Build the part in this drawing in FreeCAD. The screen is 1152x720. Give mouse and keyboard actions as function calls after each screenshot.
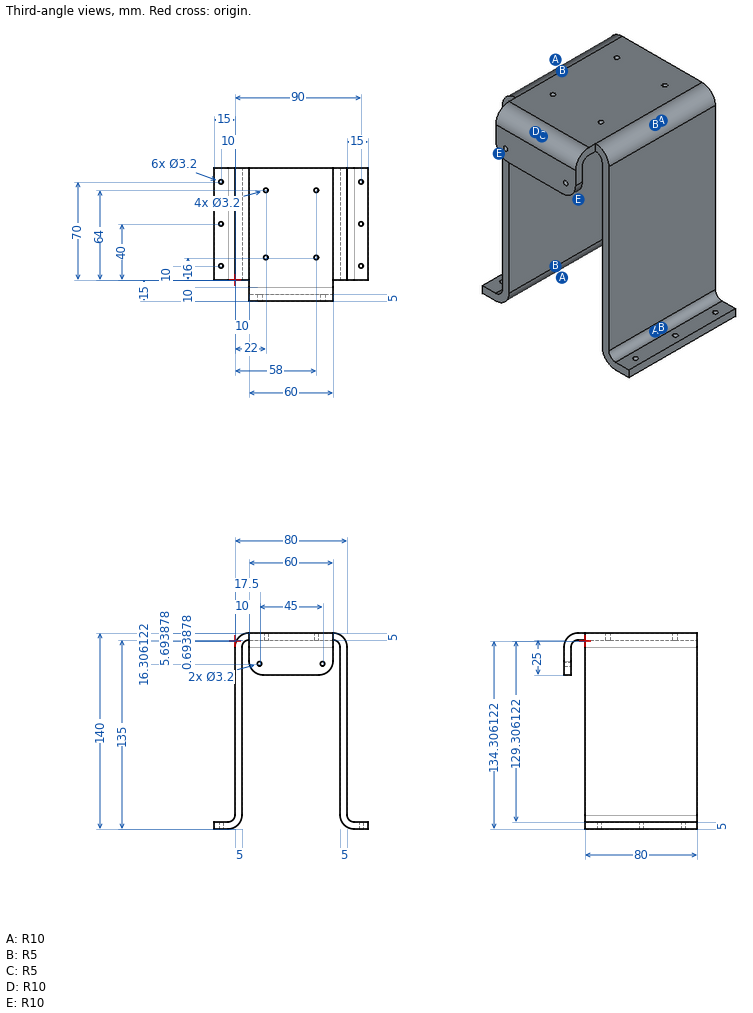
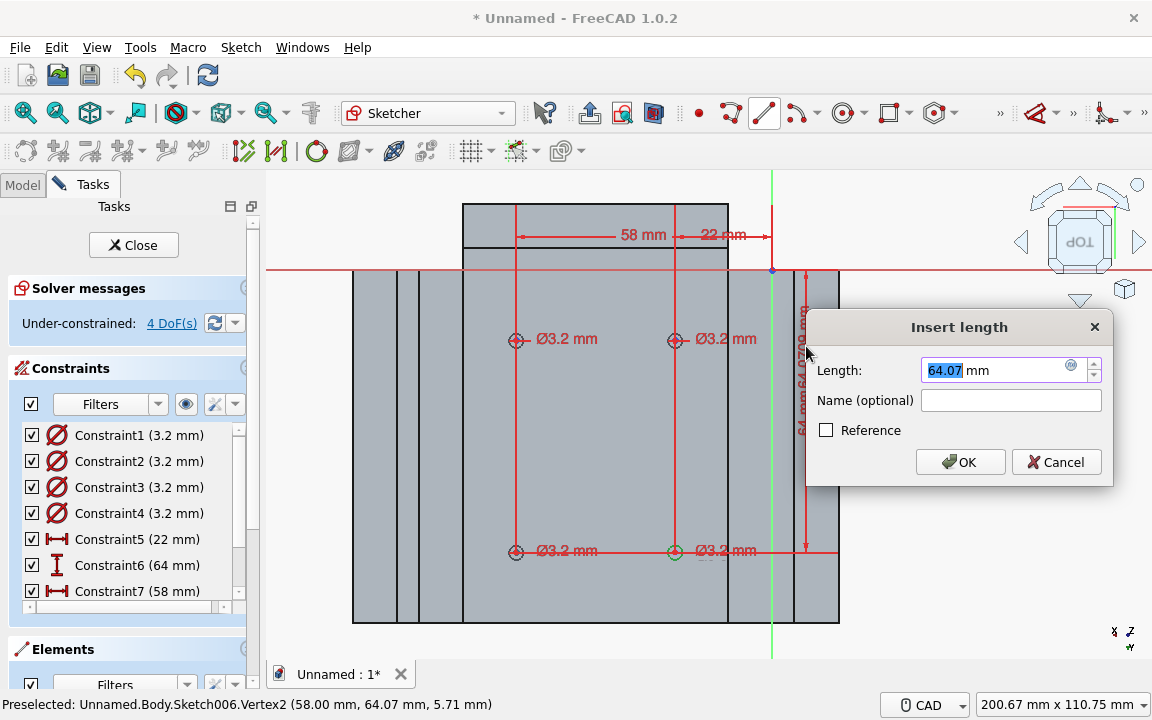
text(64)
key(Return)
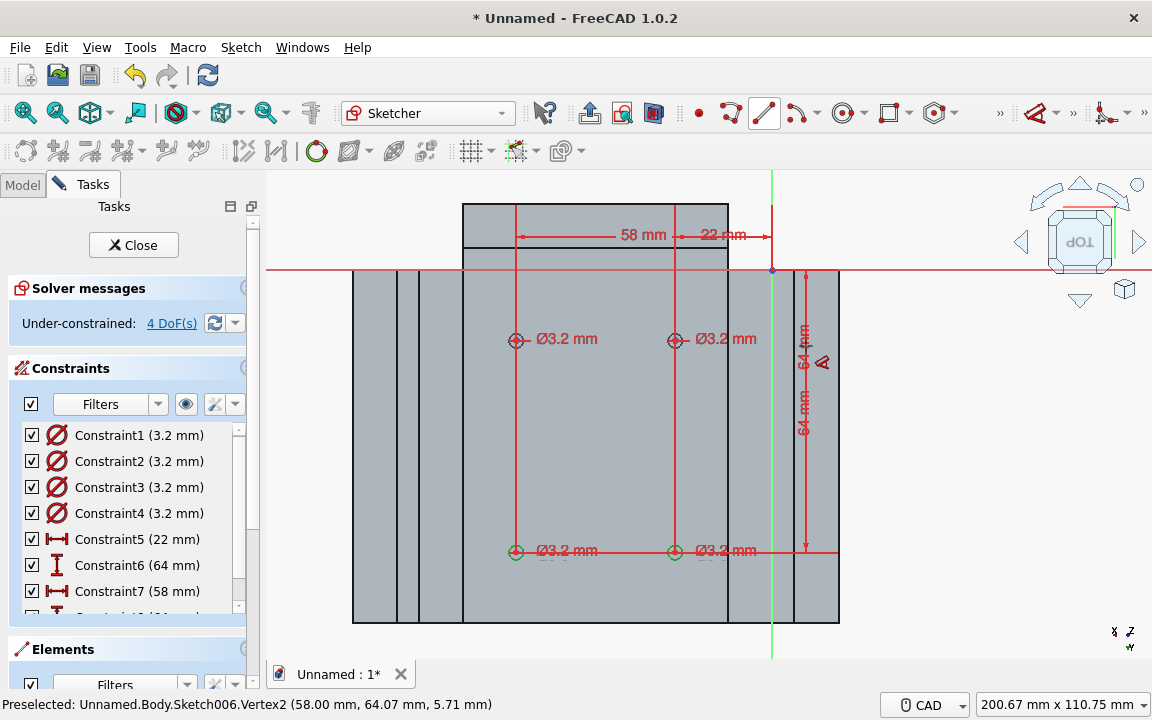
click(516, 341)
click(555, 236)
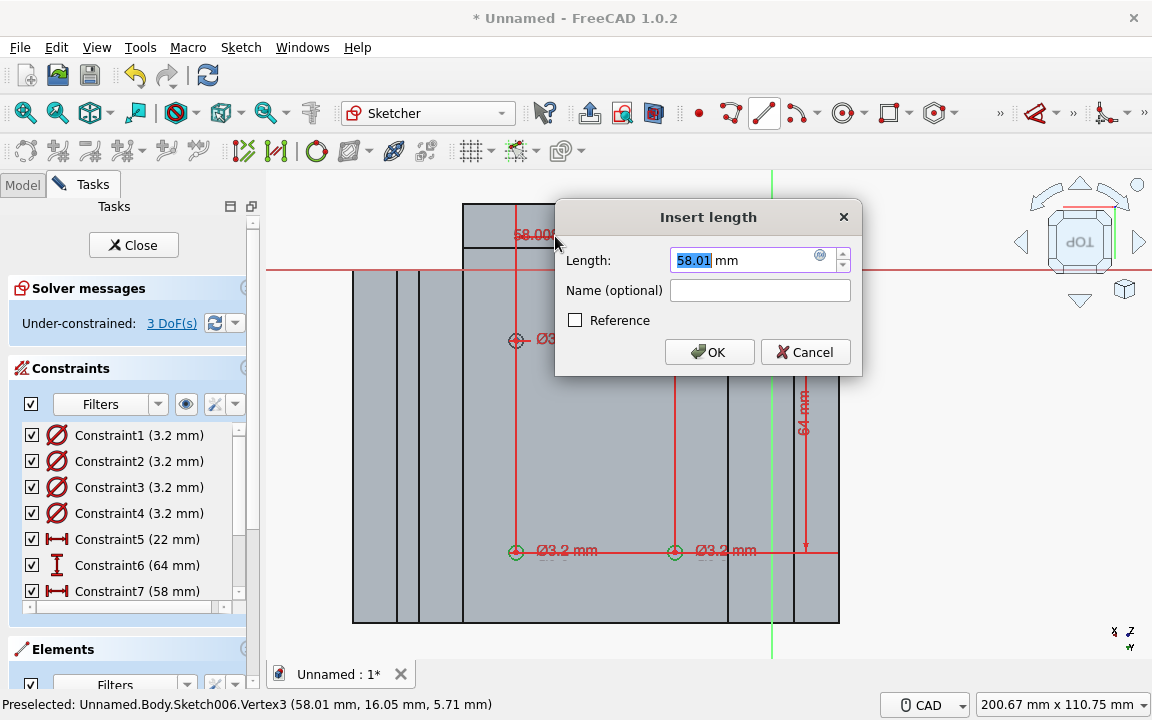
text(58)
key(Return)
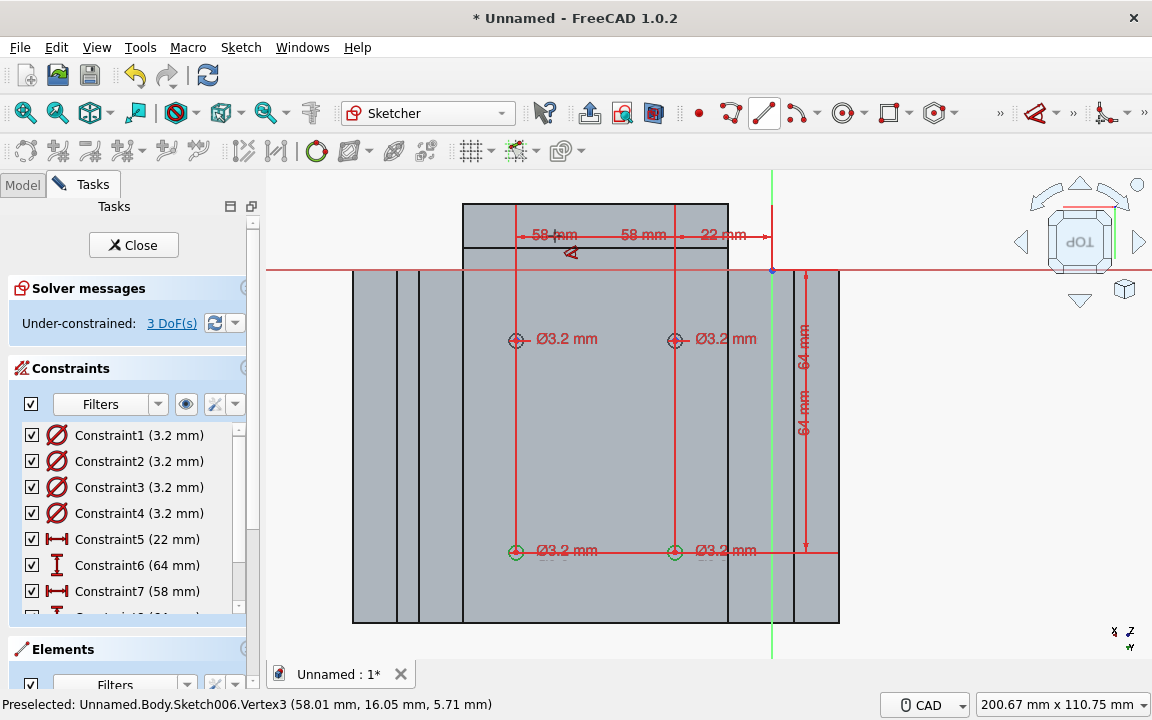
click(516, 341)
click(806, 306)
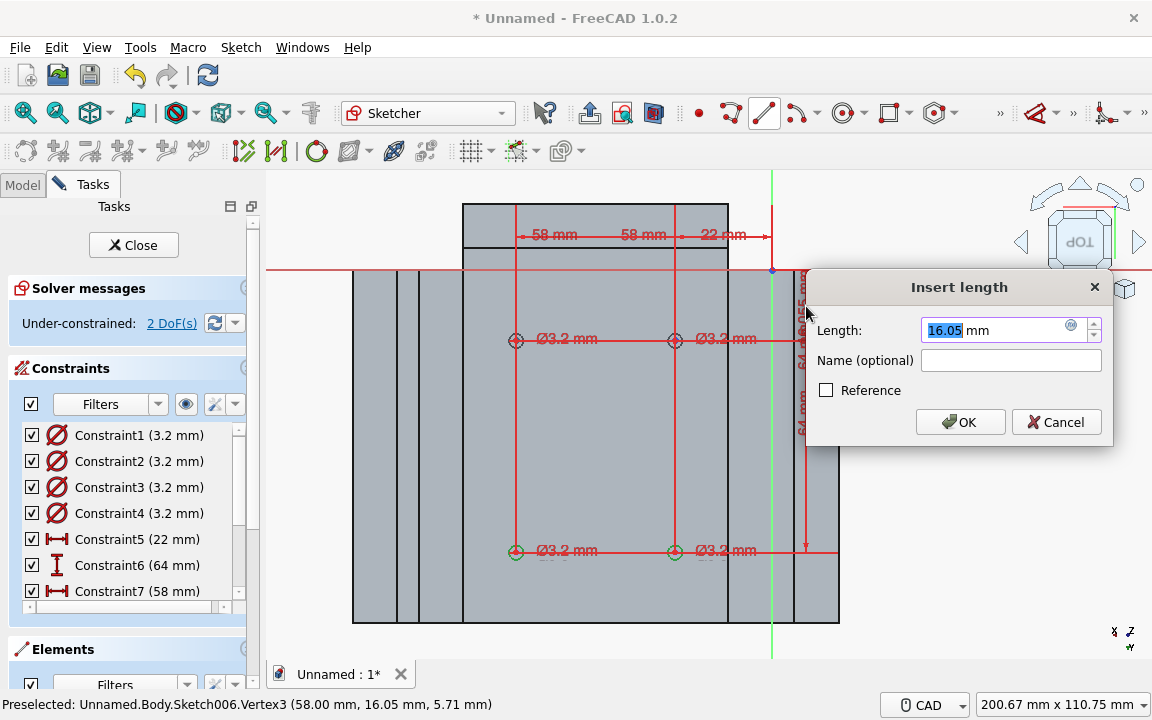
text(16)
key(Return)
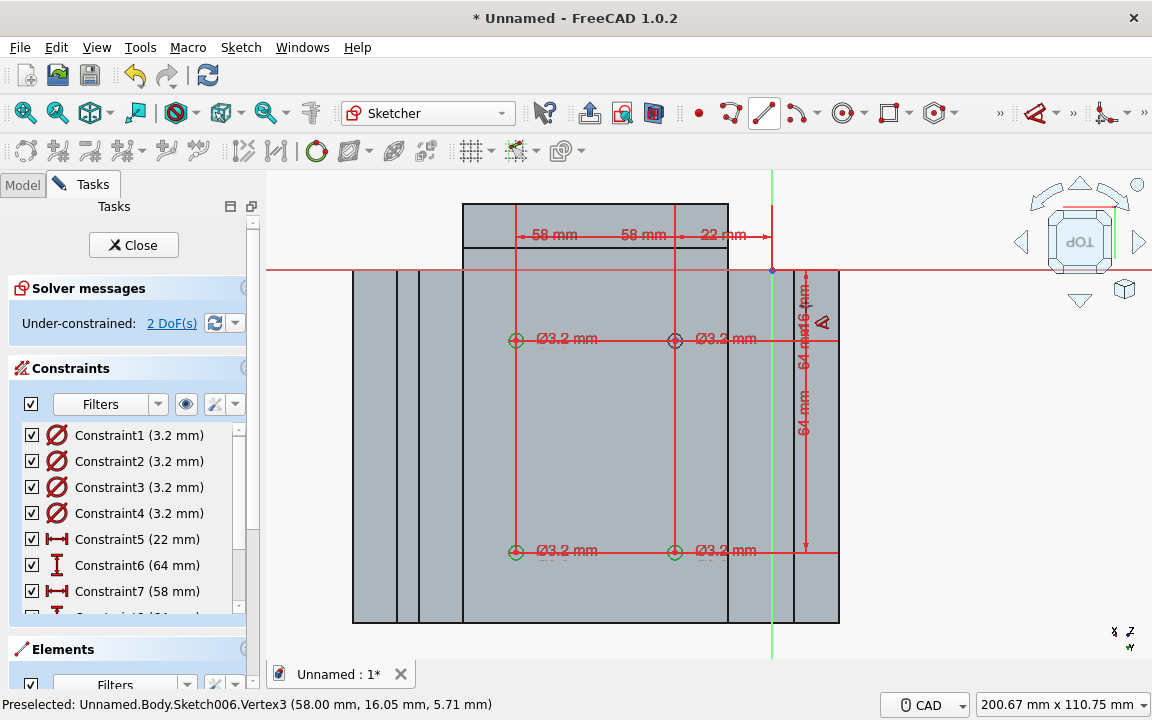
click(675, 341)
click(724, 375)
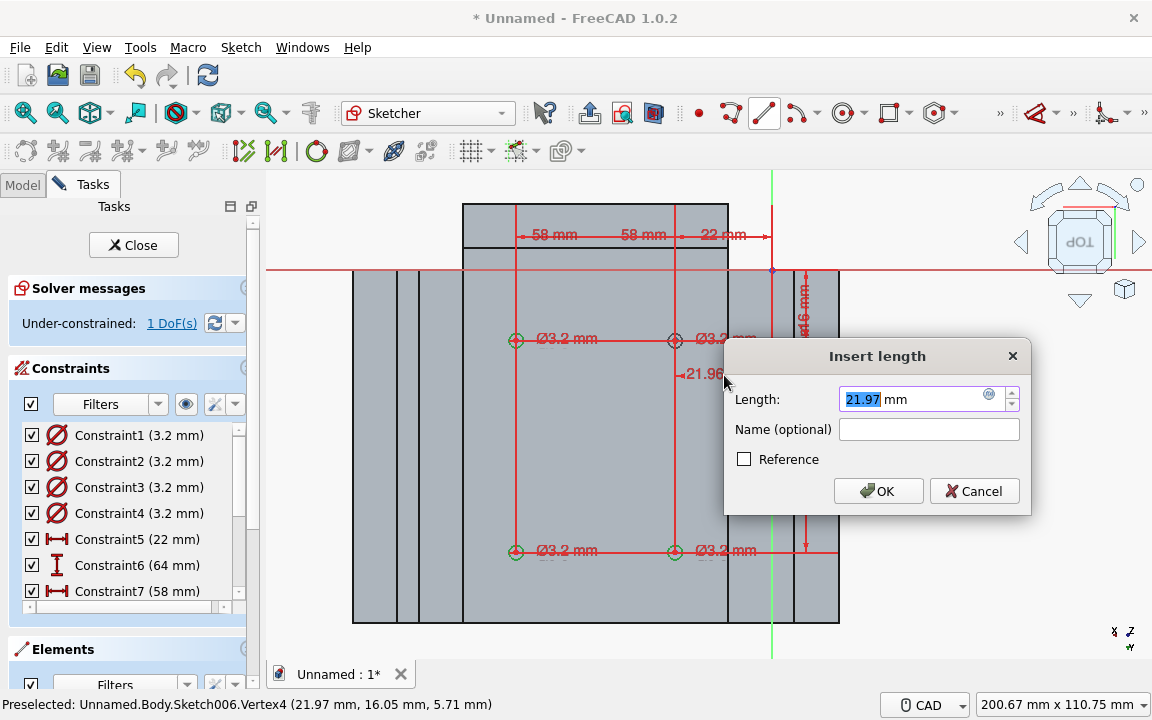
text(22)
key(Return)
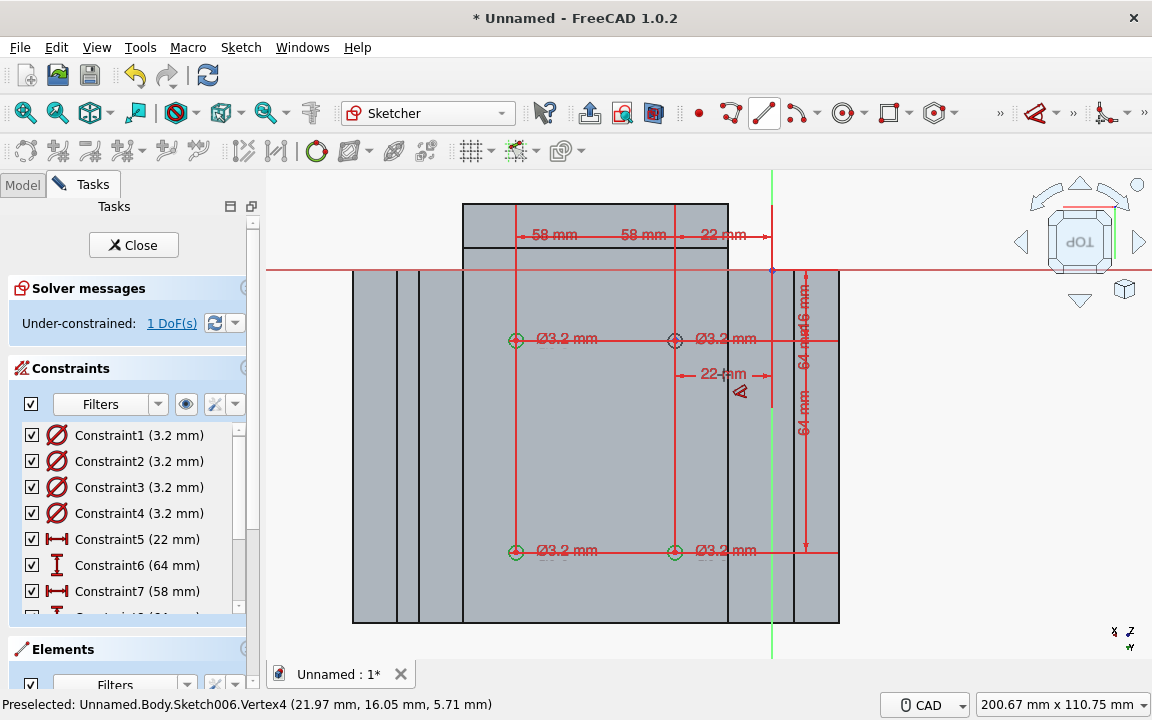
click(675, 341)
click(641, 306)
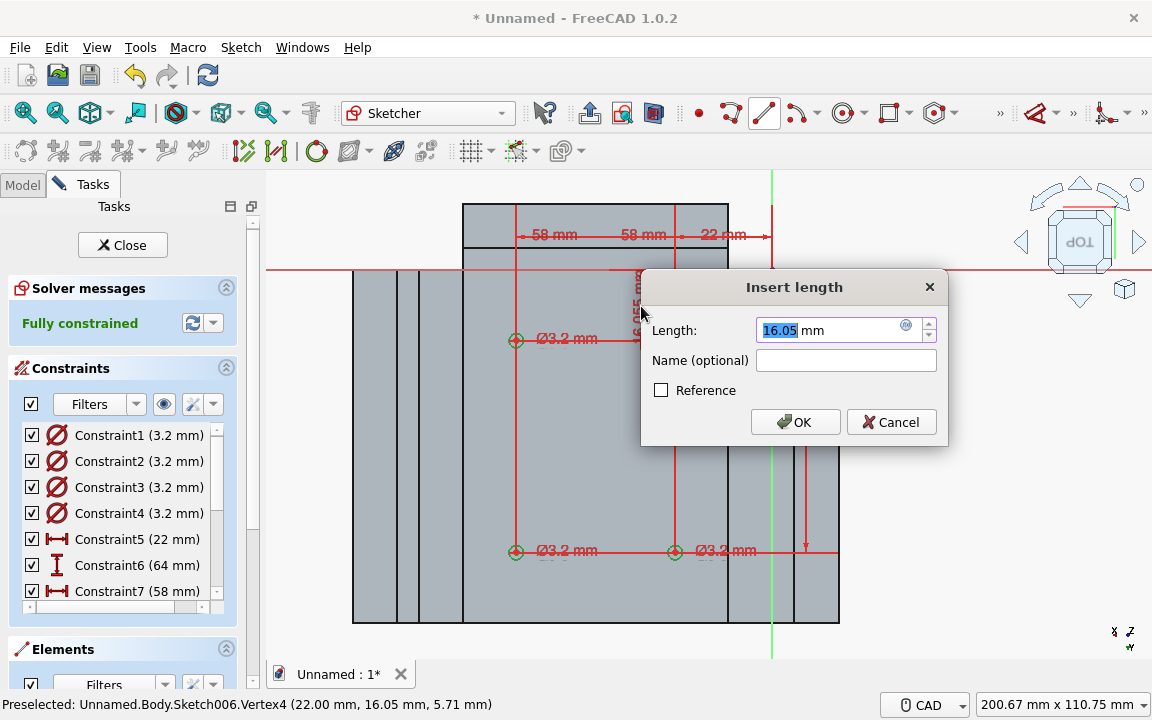
text(16)
key(Return)
key(Escape)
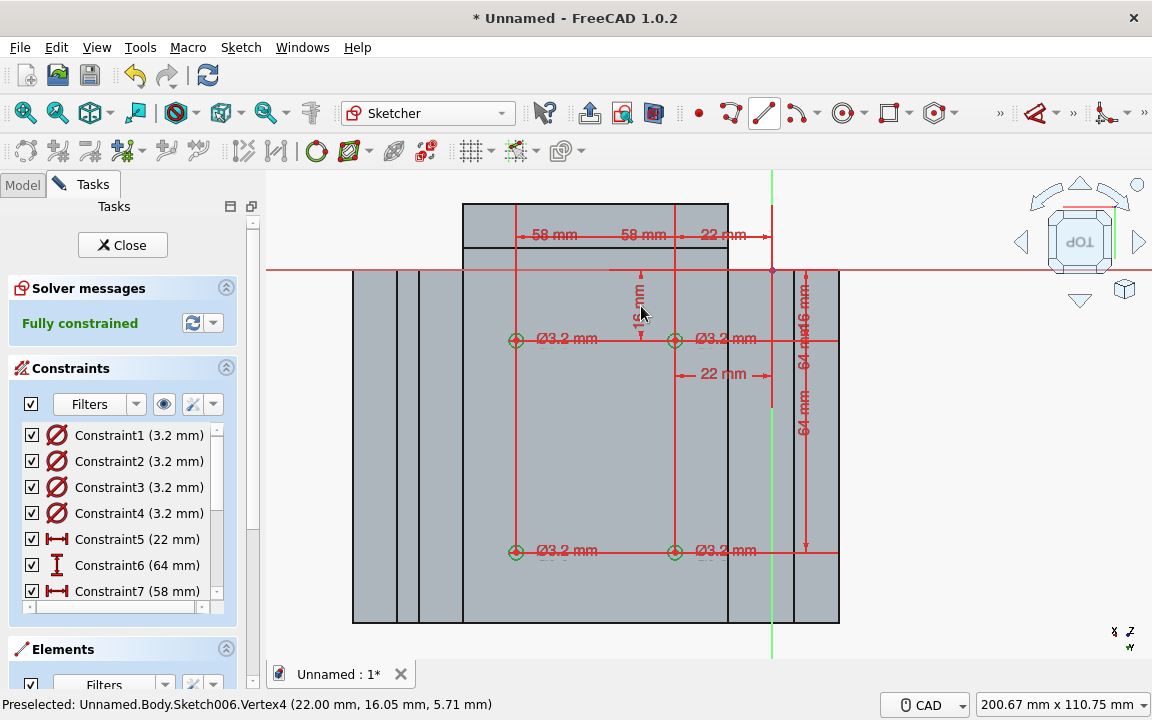
click(123, 245)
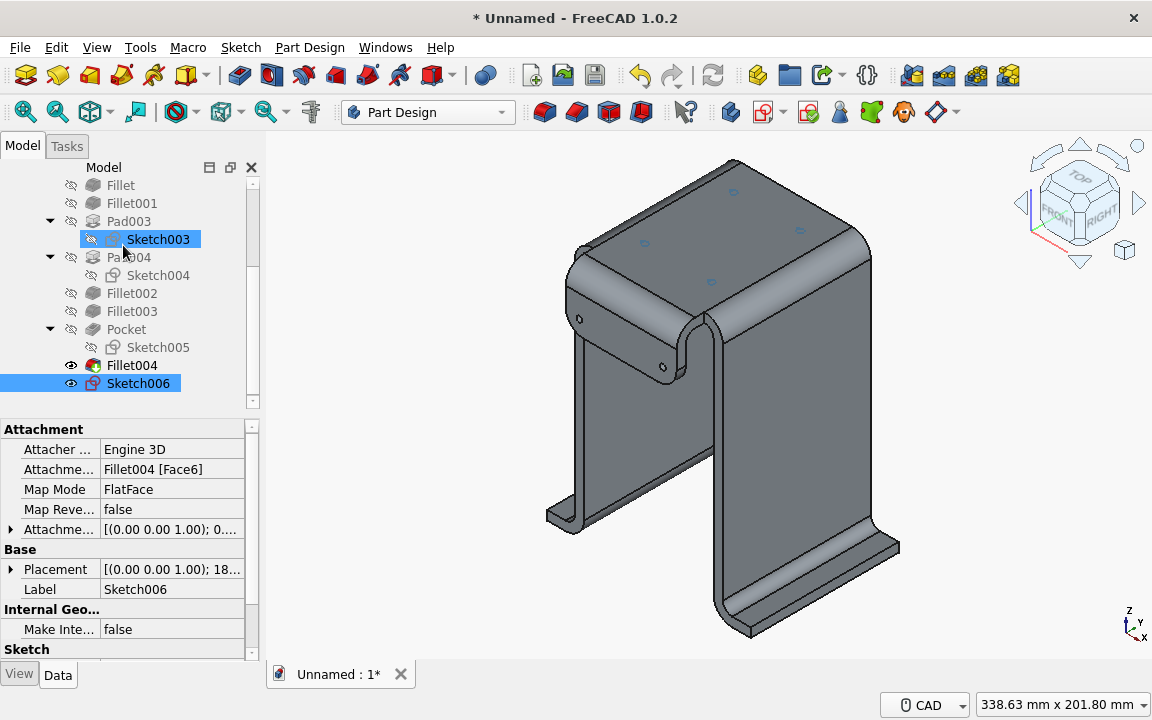
click(240, 76)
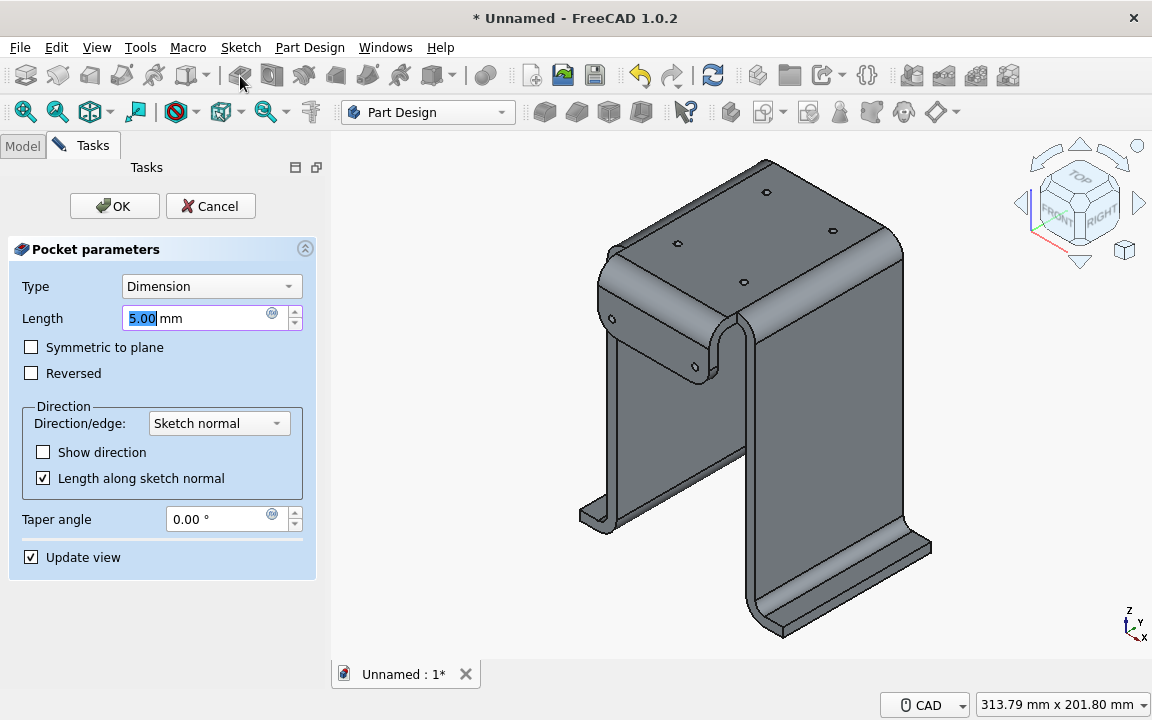
click(212, 286)